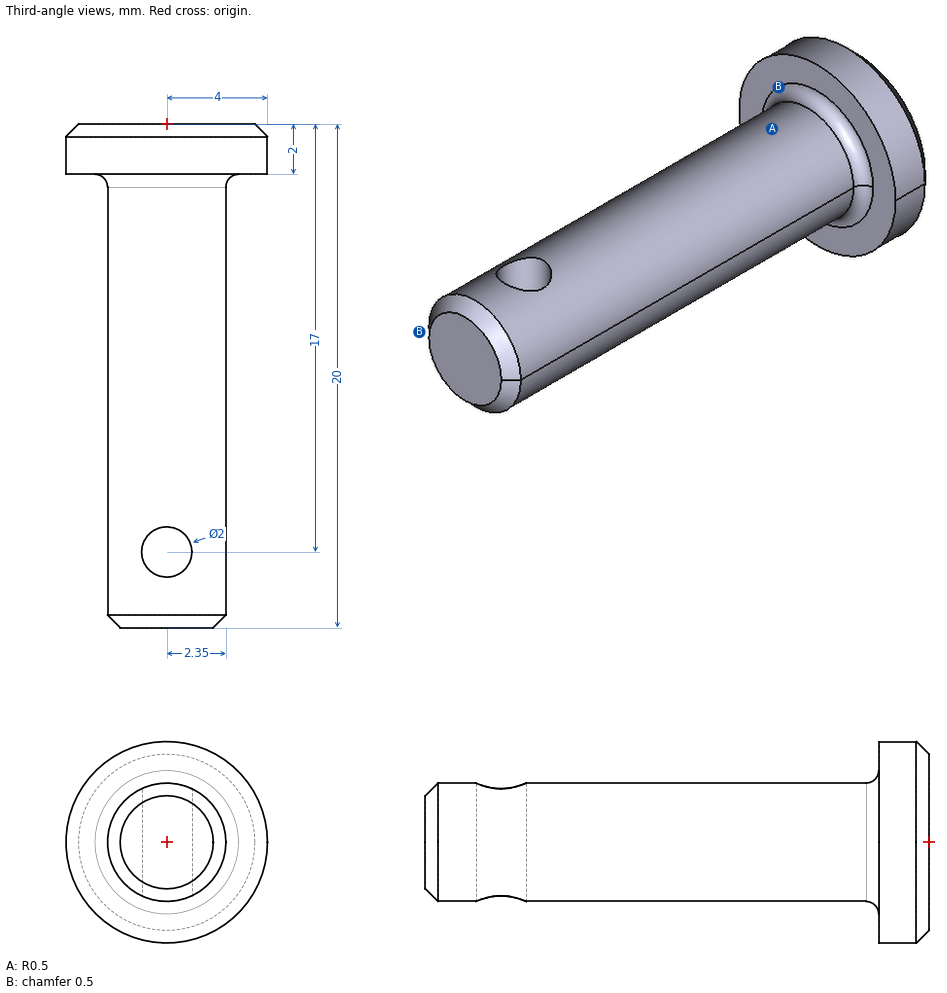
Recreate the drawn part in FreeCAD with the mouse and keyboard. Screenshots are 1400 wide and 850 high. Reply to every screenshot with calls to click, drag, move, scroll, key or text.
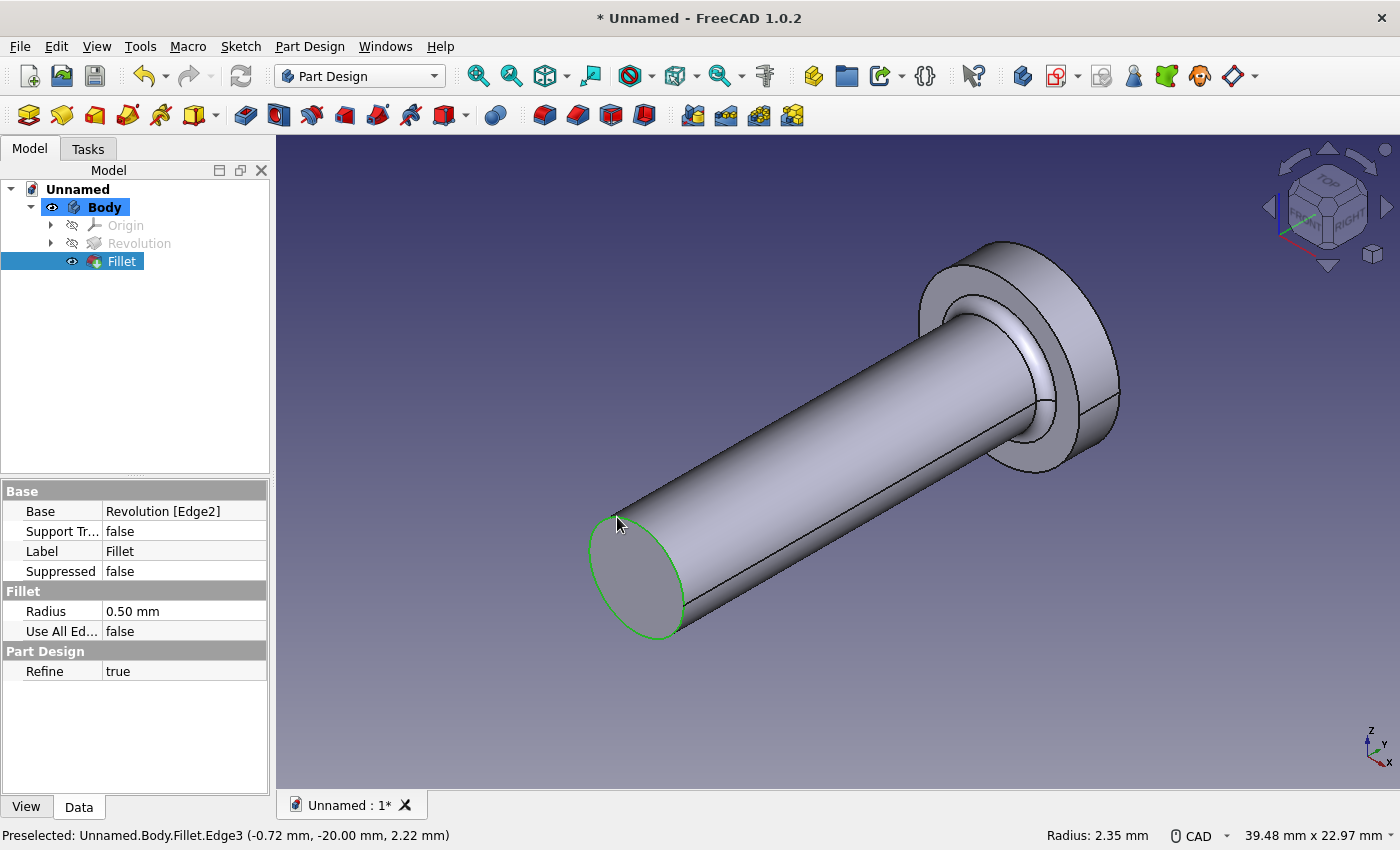
key(2)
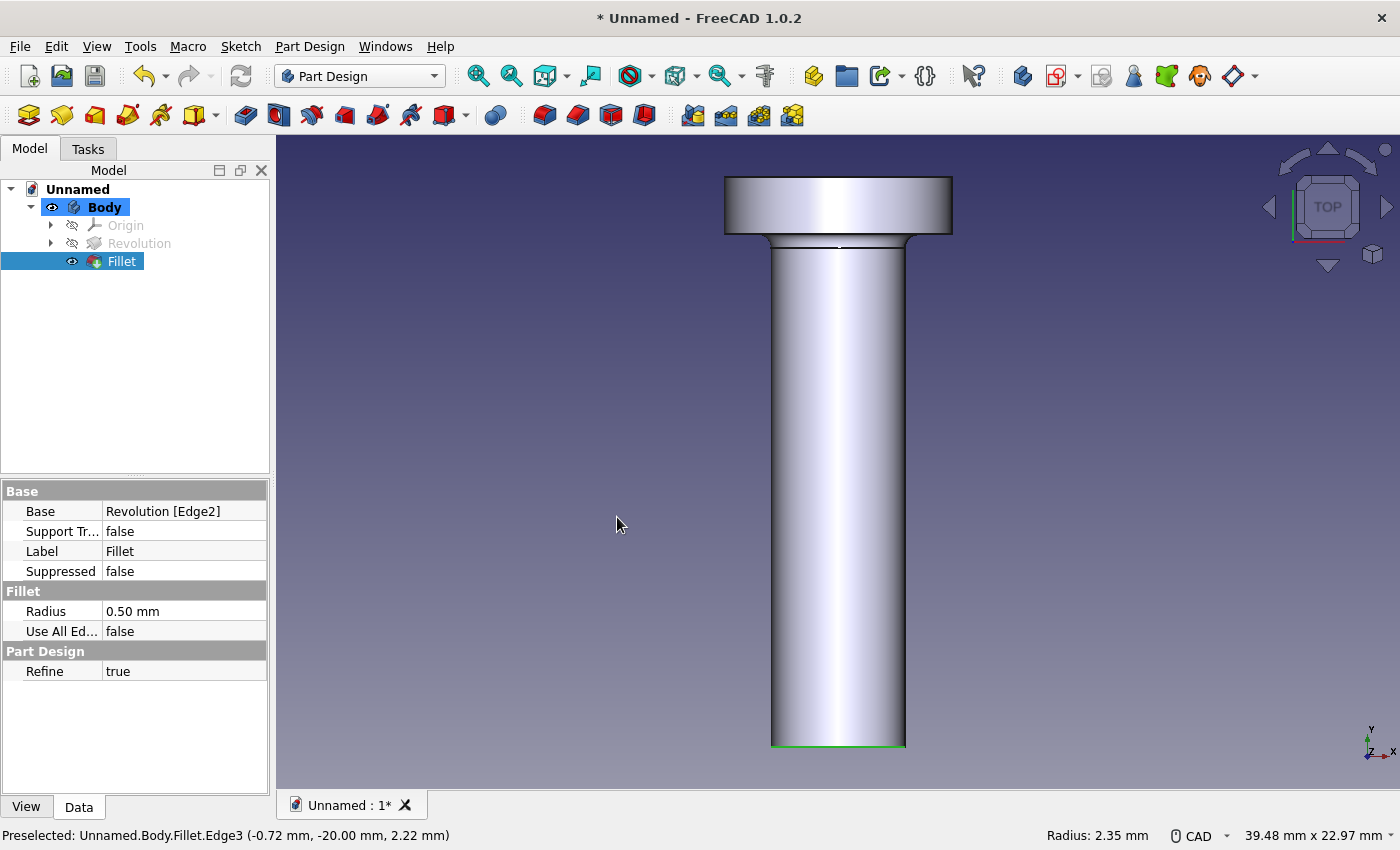
click(746, 176, ctrl)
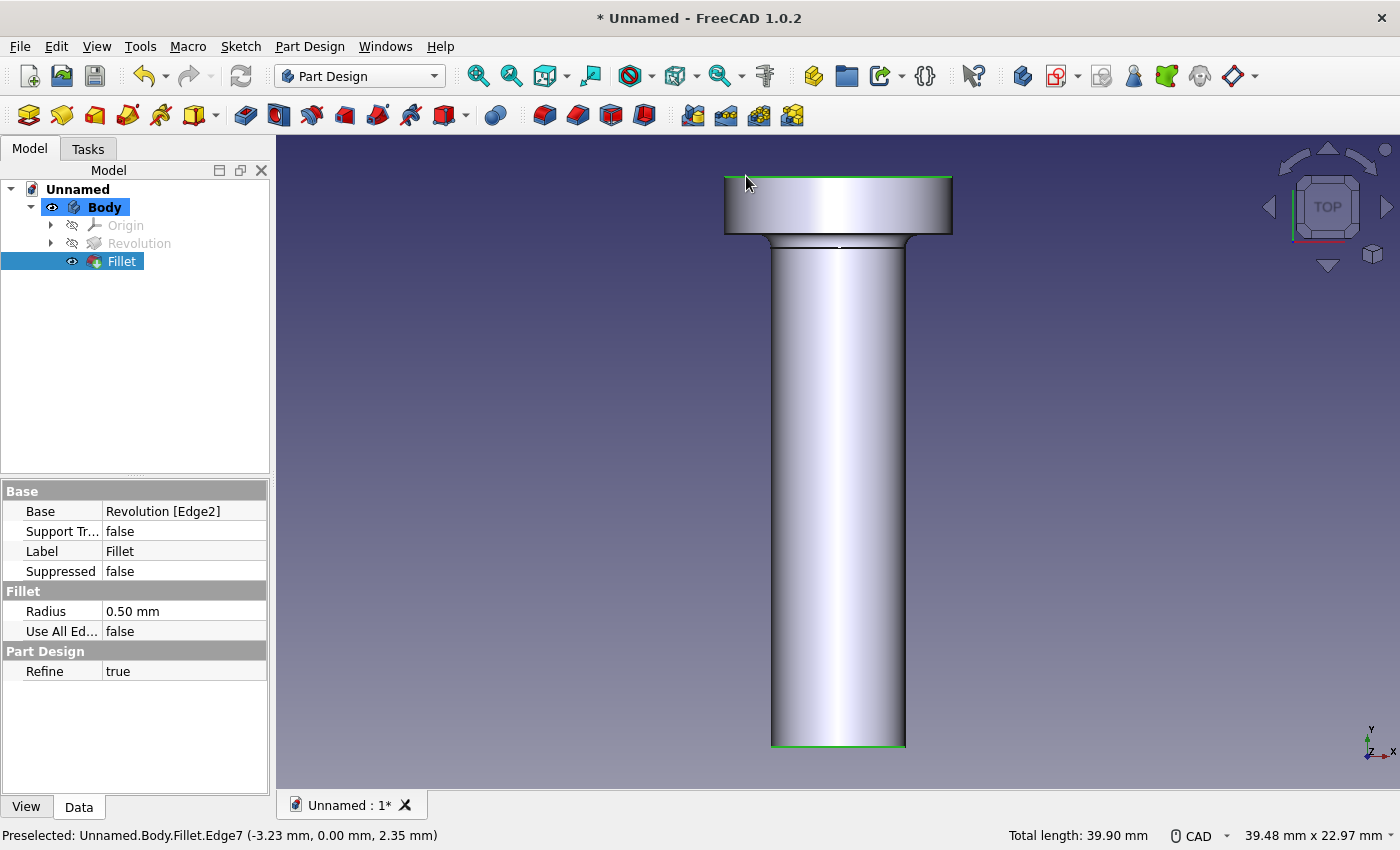
click(578, 116)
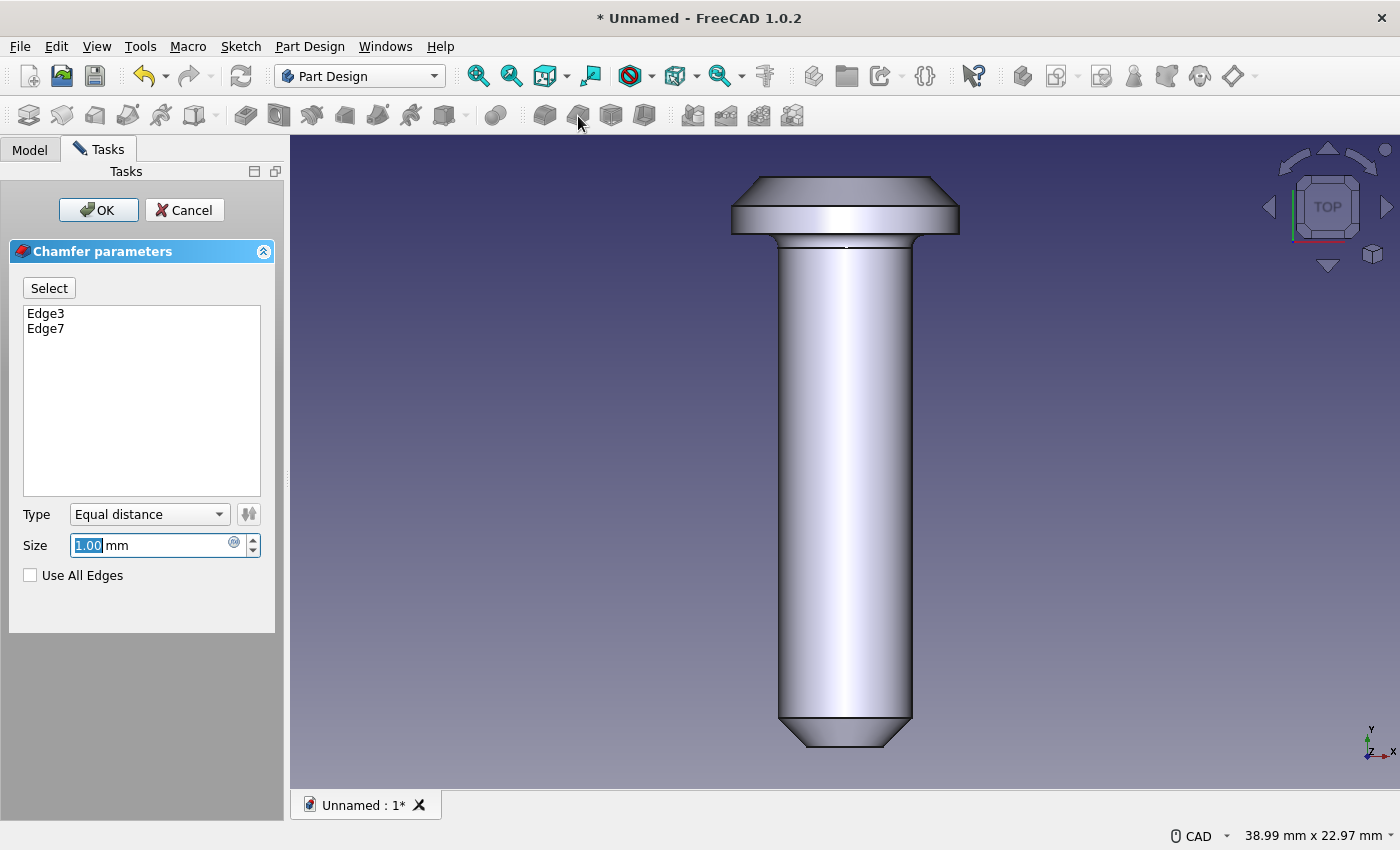
text(0.5)
key(Tab)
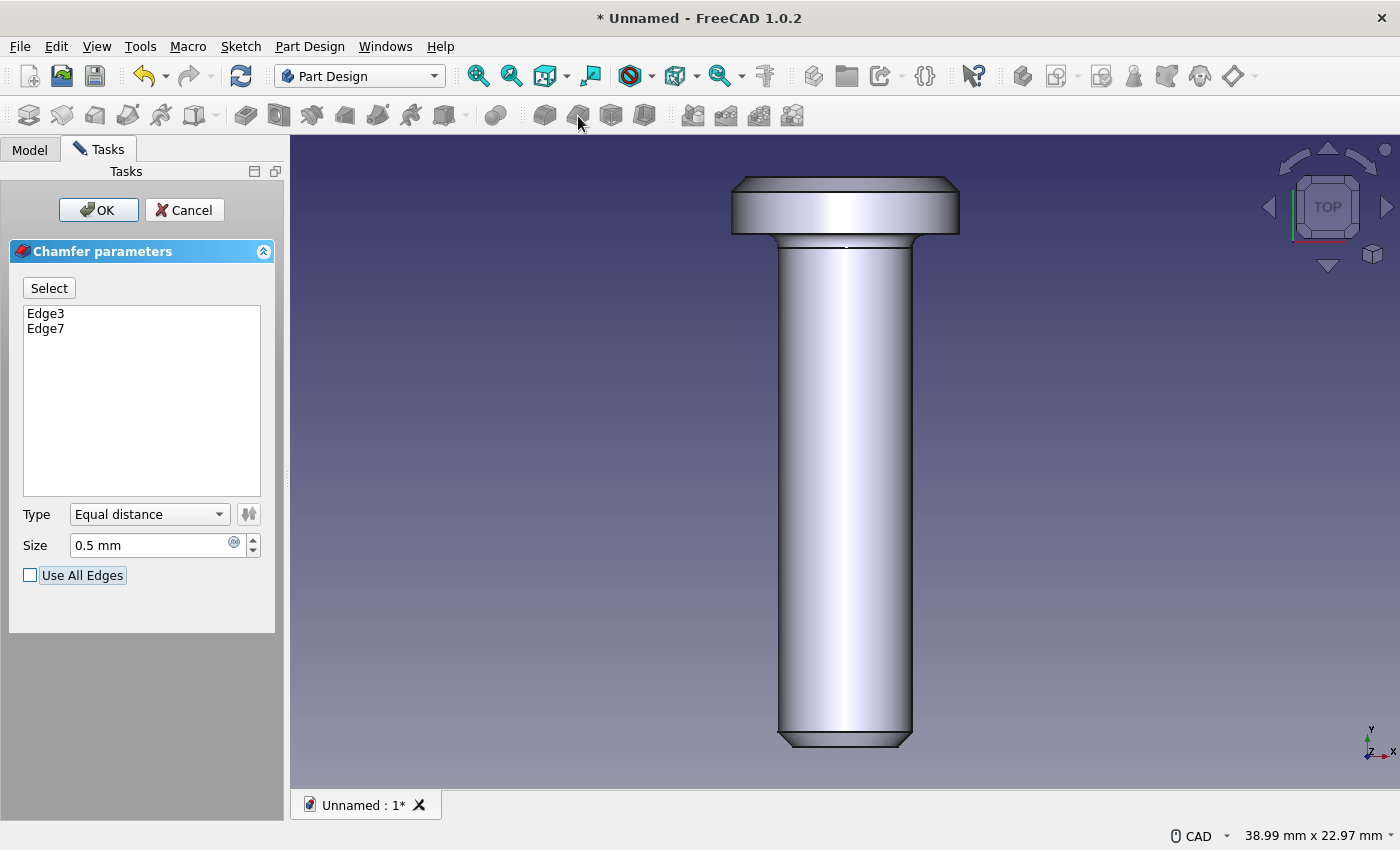
click(99, 210)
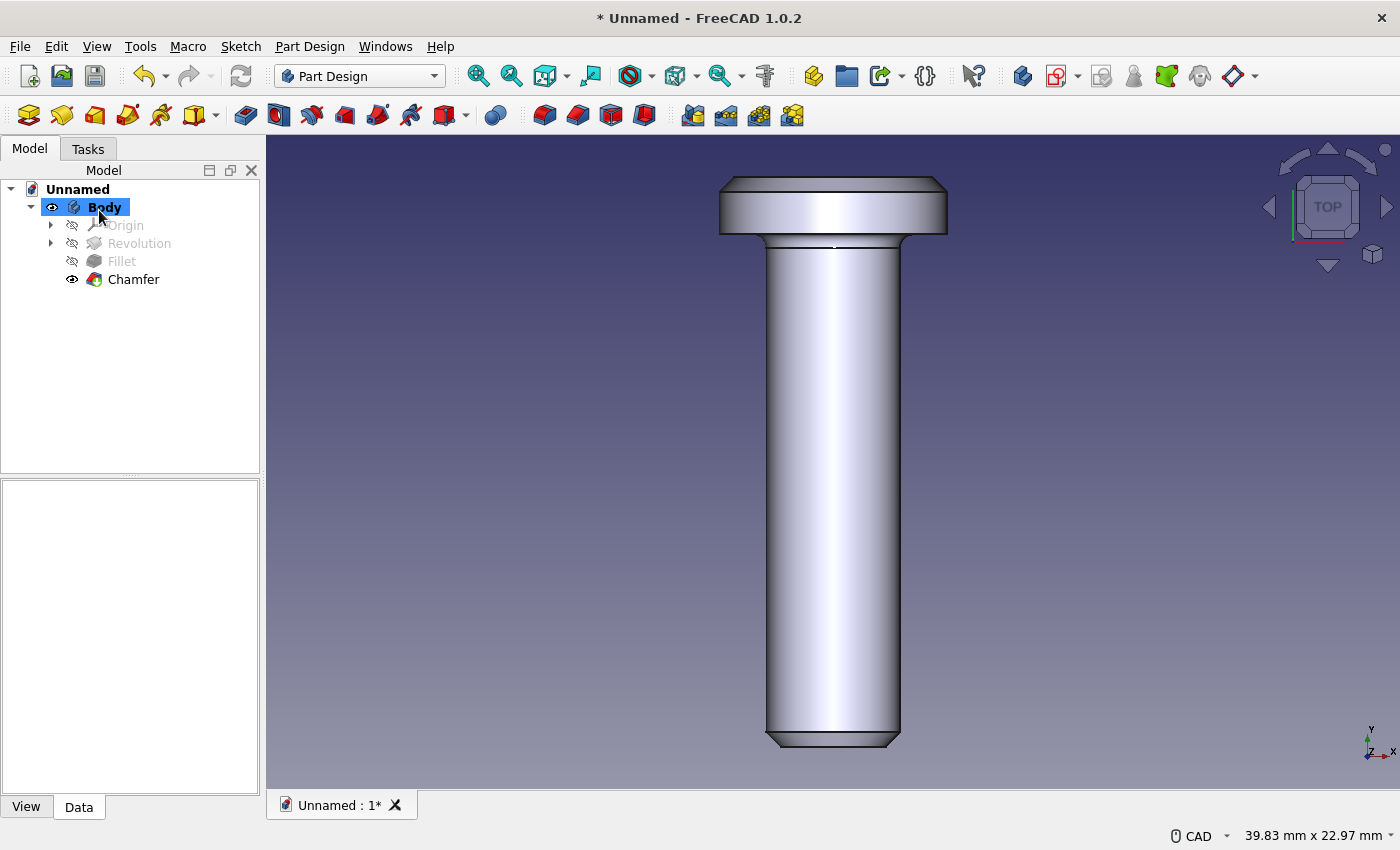
click(1056, 76)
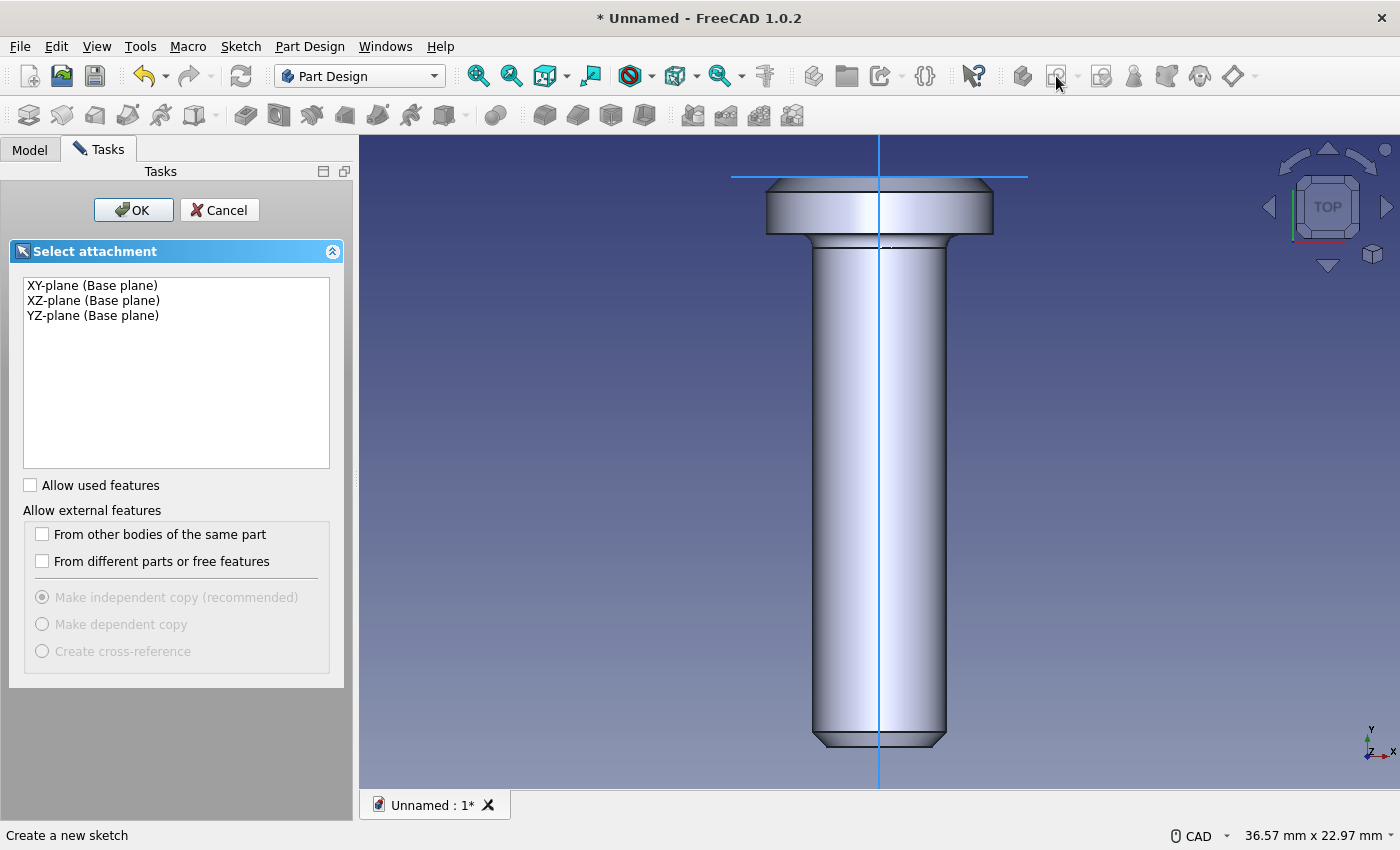
click(84, 286)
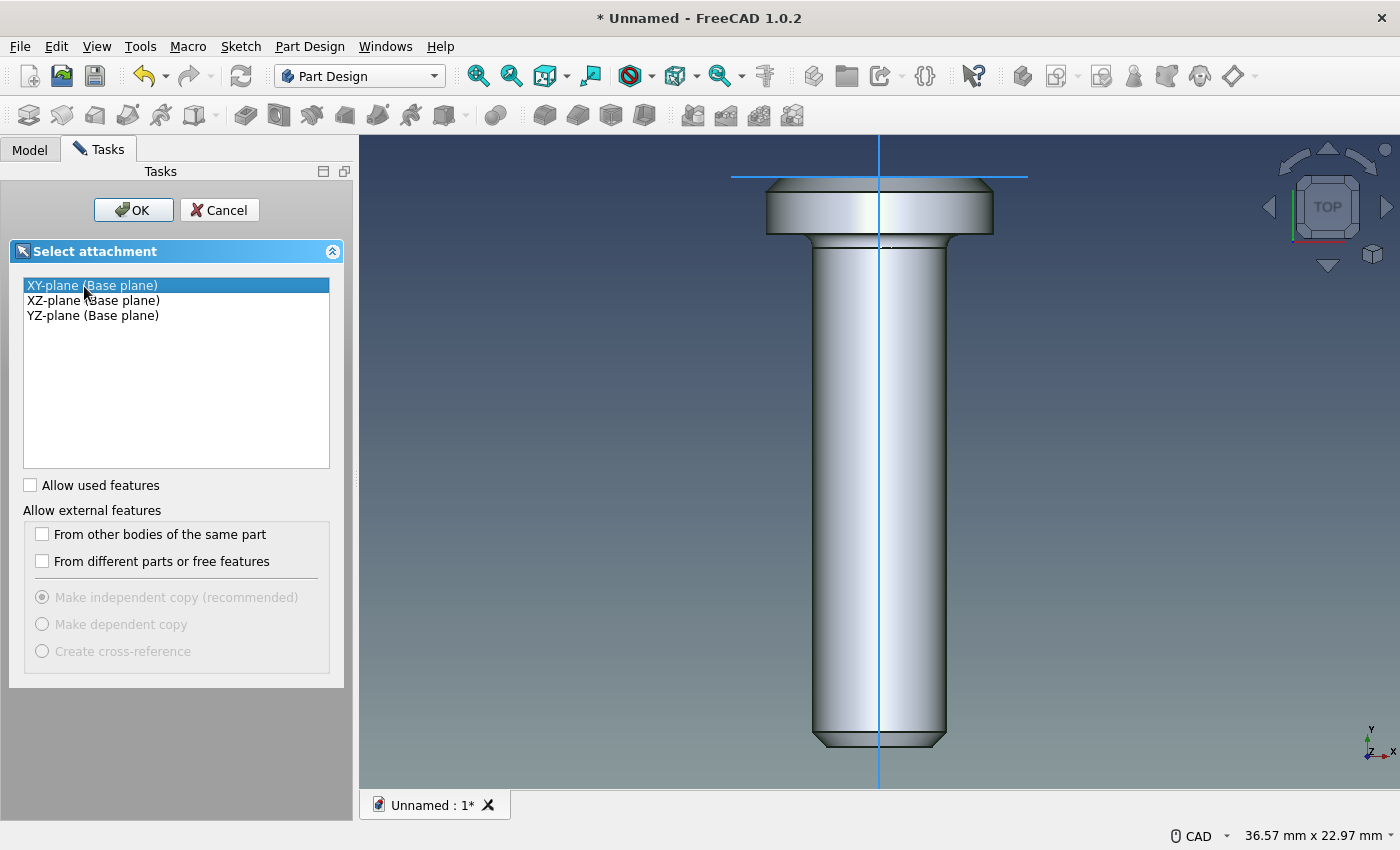
click(134, 210)